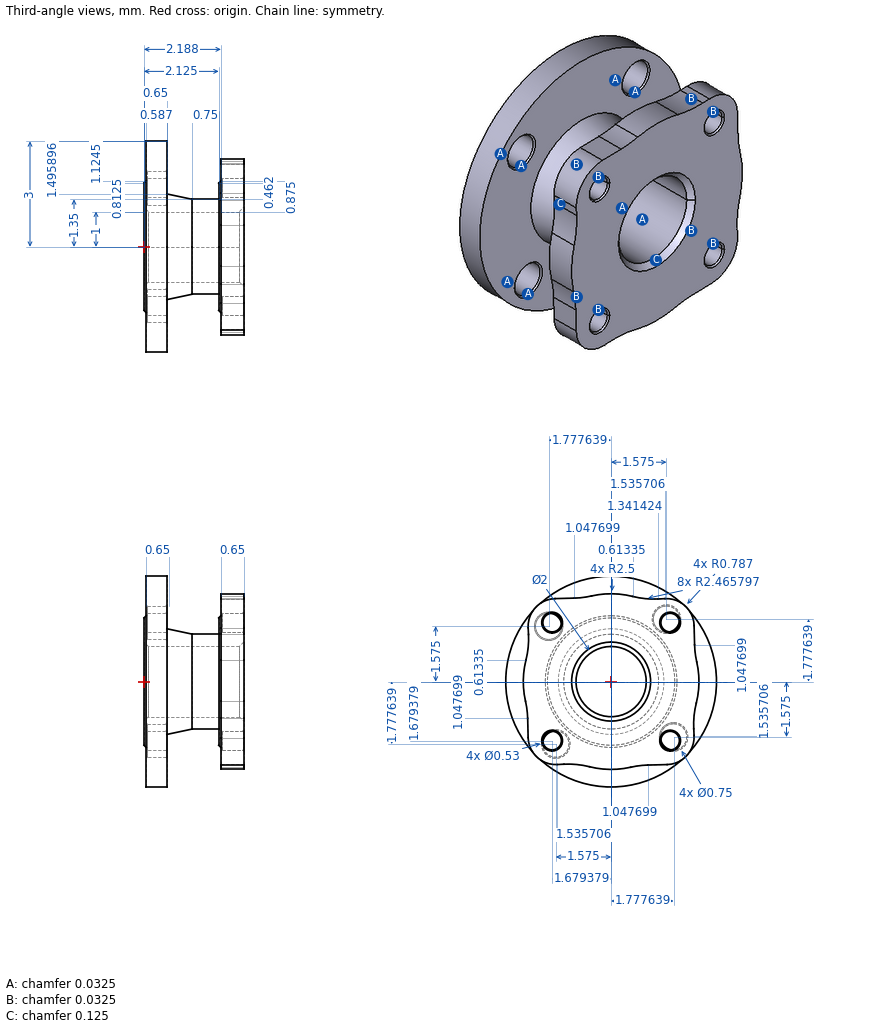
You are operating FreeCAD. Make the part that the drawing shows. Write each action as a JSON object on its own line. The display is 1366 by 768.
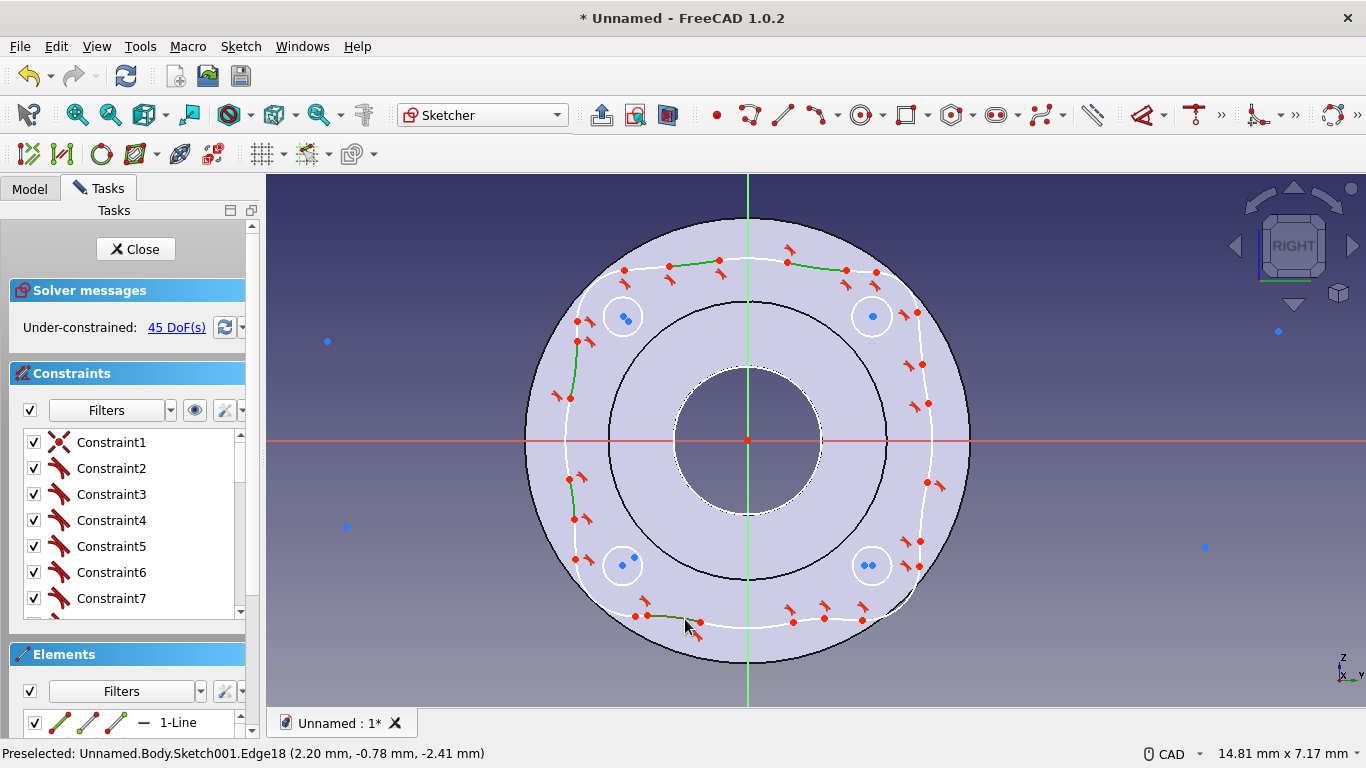
{"action": "scroll", "coordinate": [815, 619], "scroll_direction": "up", "scroll_amount": 2}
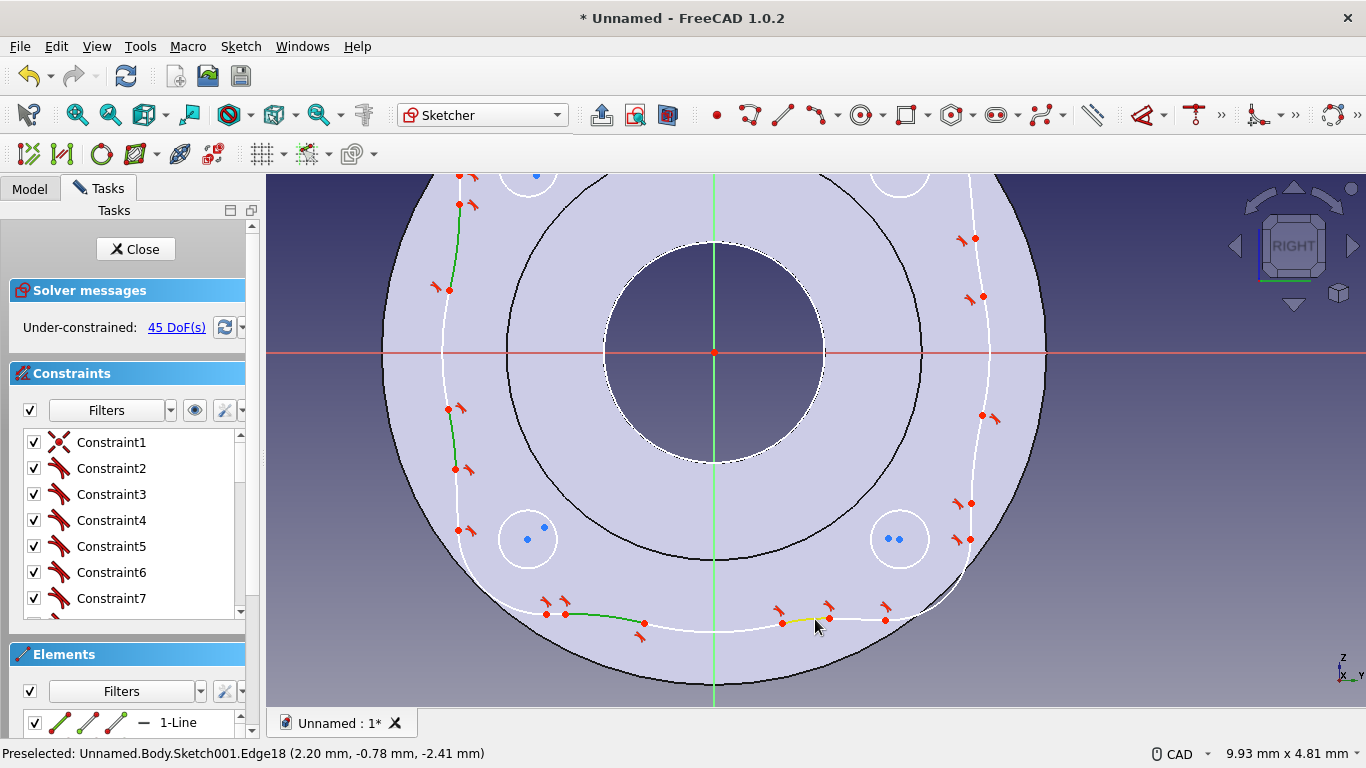
{"action": "left_click", "coordinate": [815, 619]}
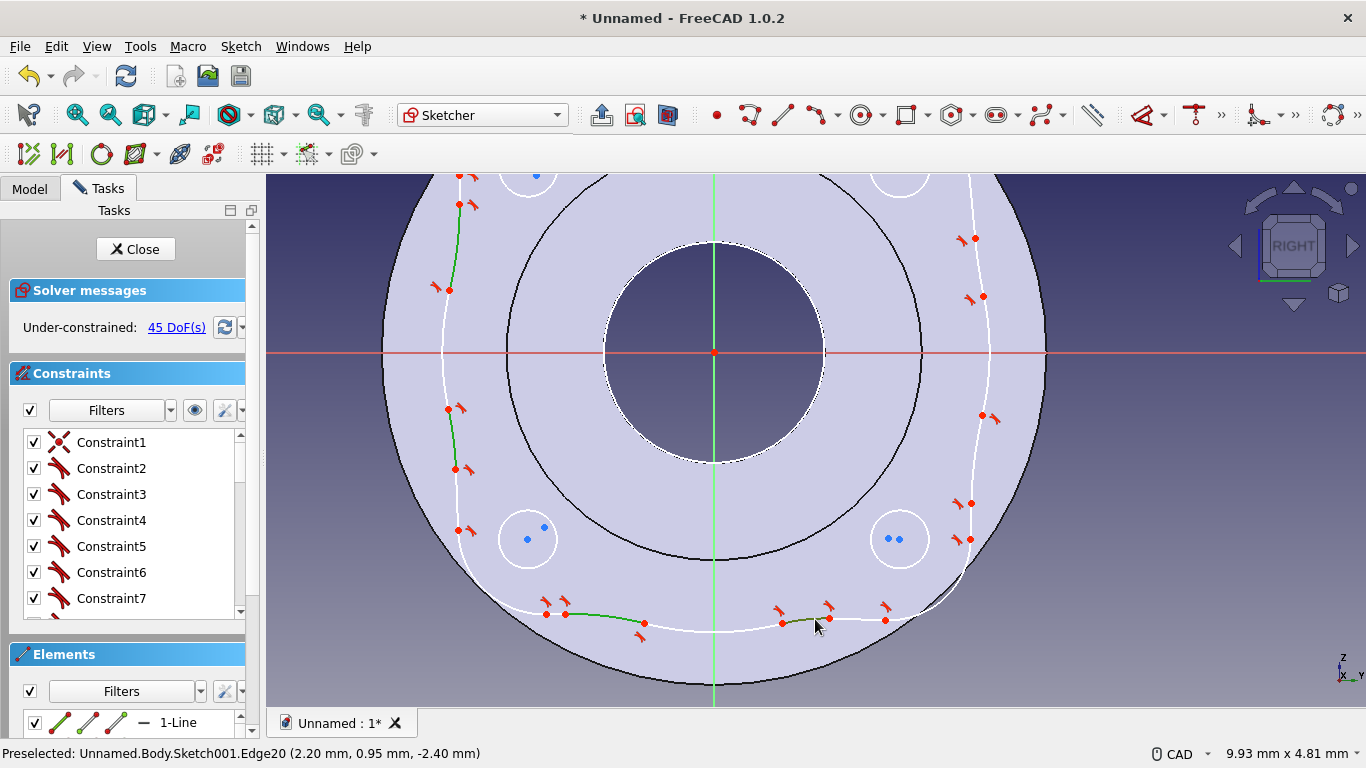
{"action": "left_click", "coordinate": [977, 441]}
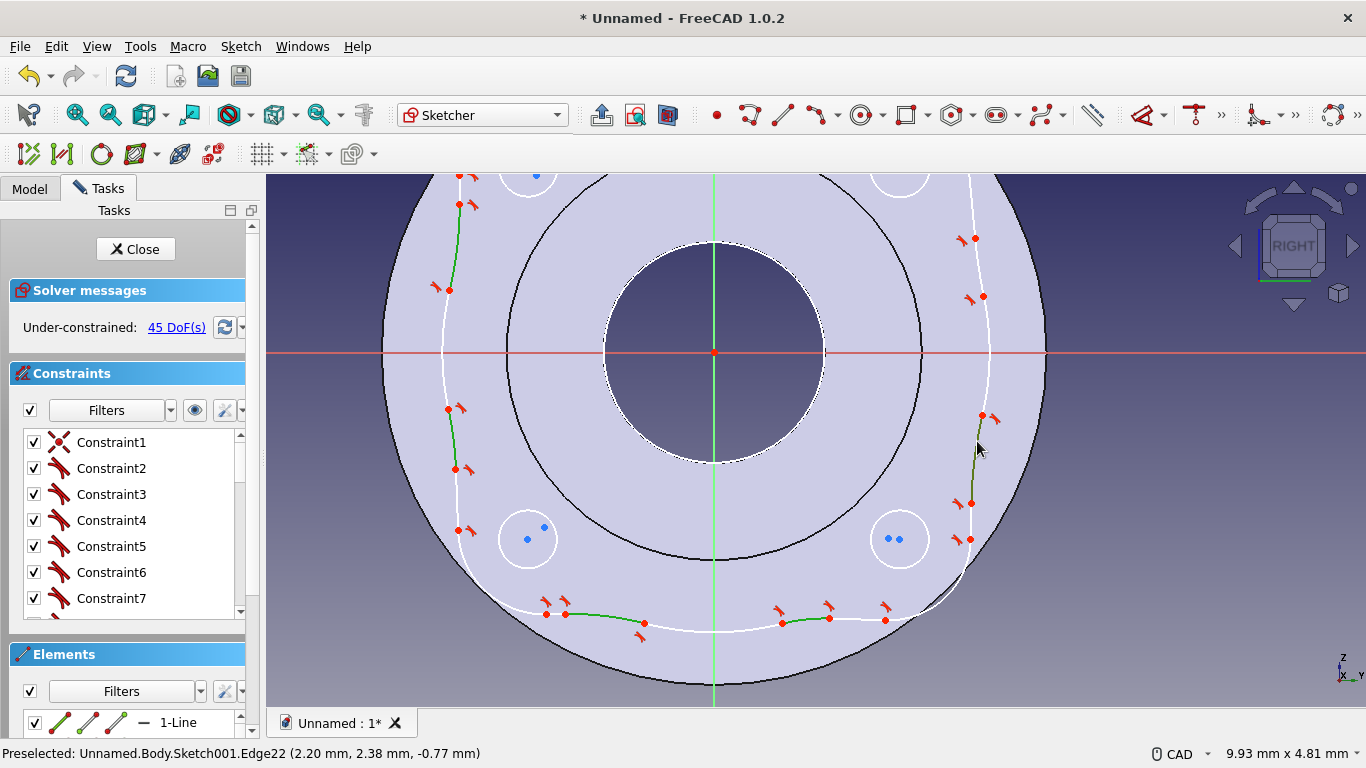
{"action": "left_click", "coordinate": [977, 256]}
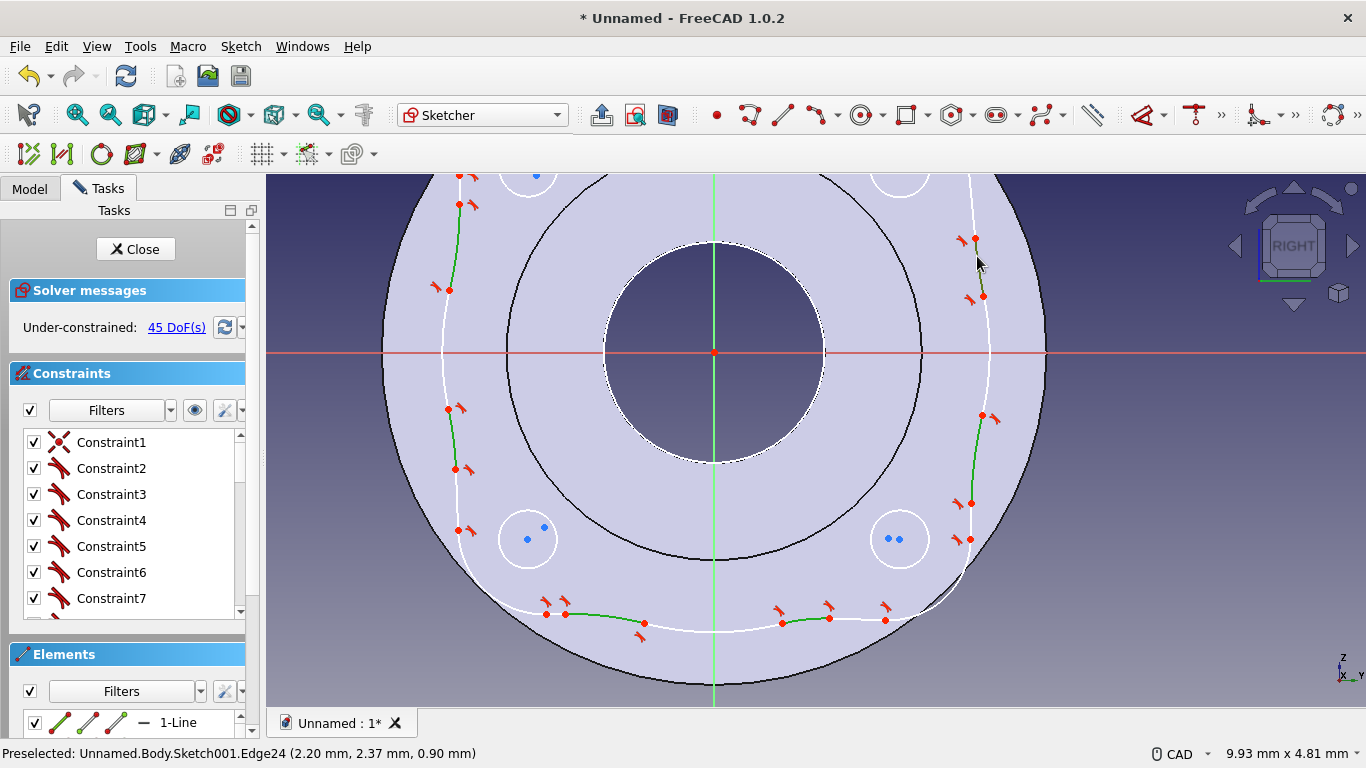
{"action": "key", "text": "e"}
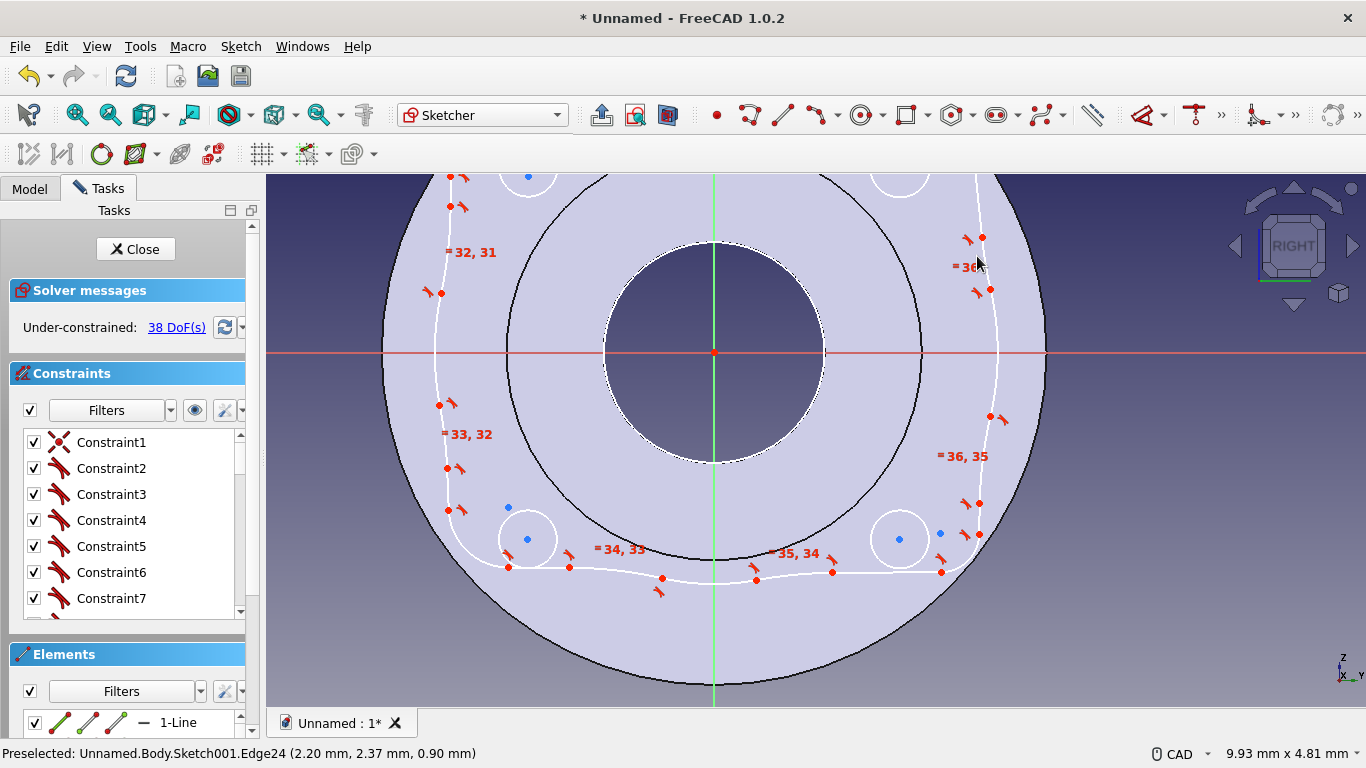
{"action": "scroll", "coordinate": [815, 619], "scroll_direction": "down", "scroll_amount": 2}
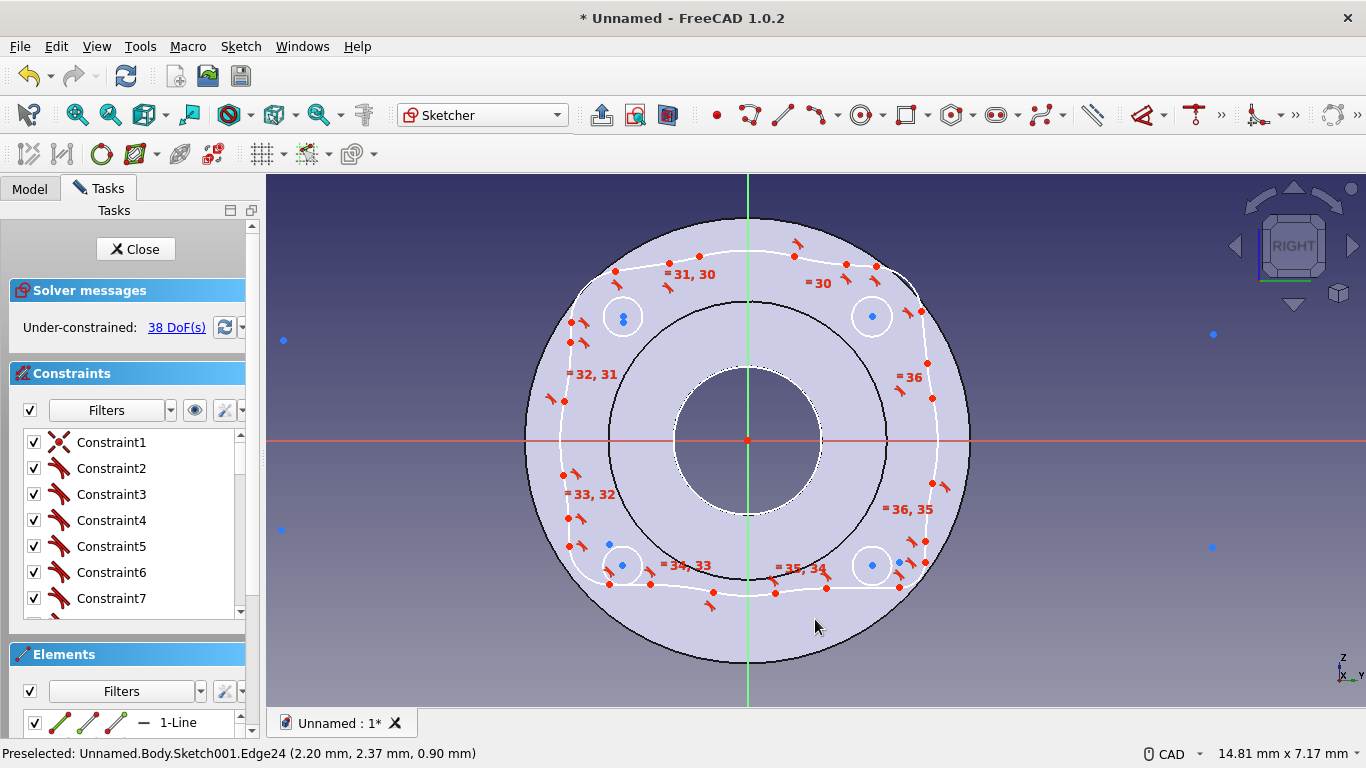
{"action": "left_click", "coordinate": [915, 292]}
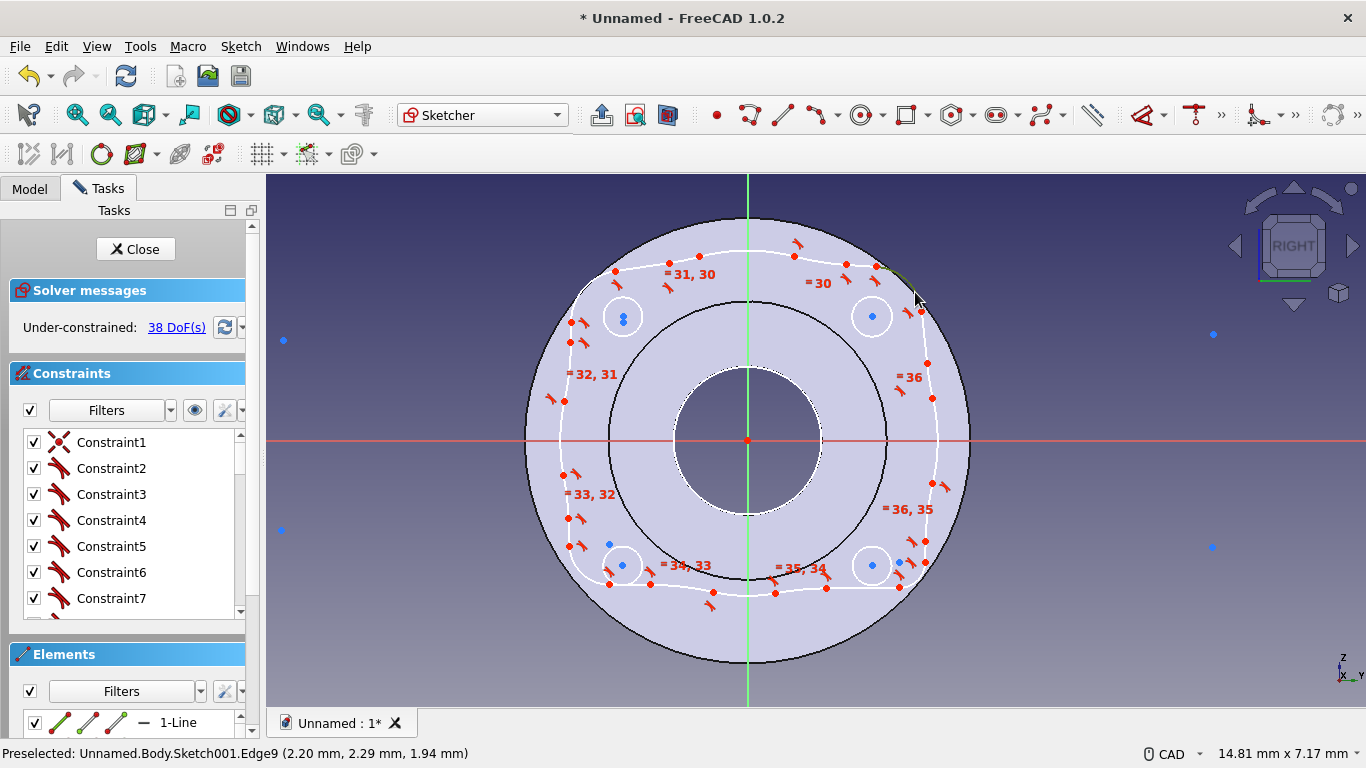
{"action": "left_click", "coordinate": [595, 279]}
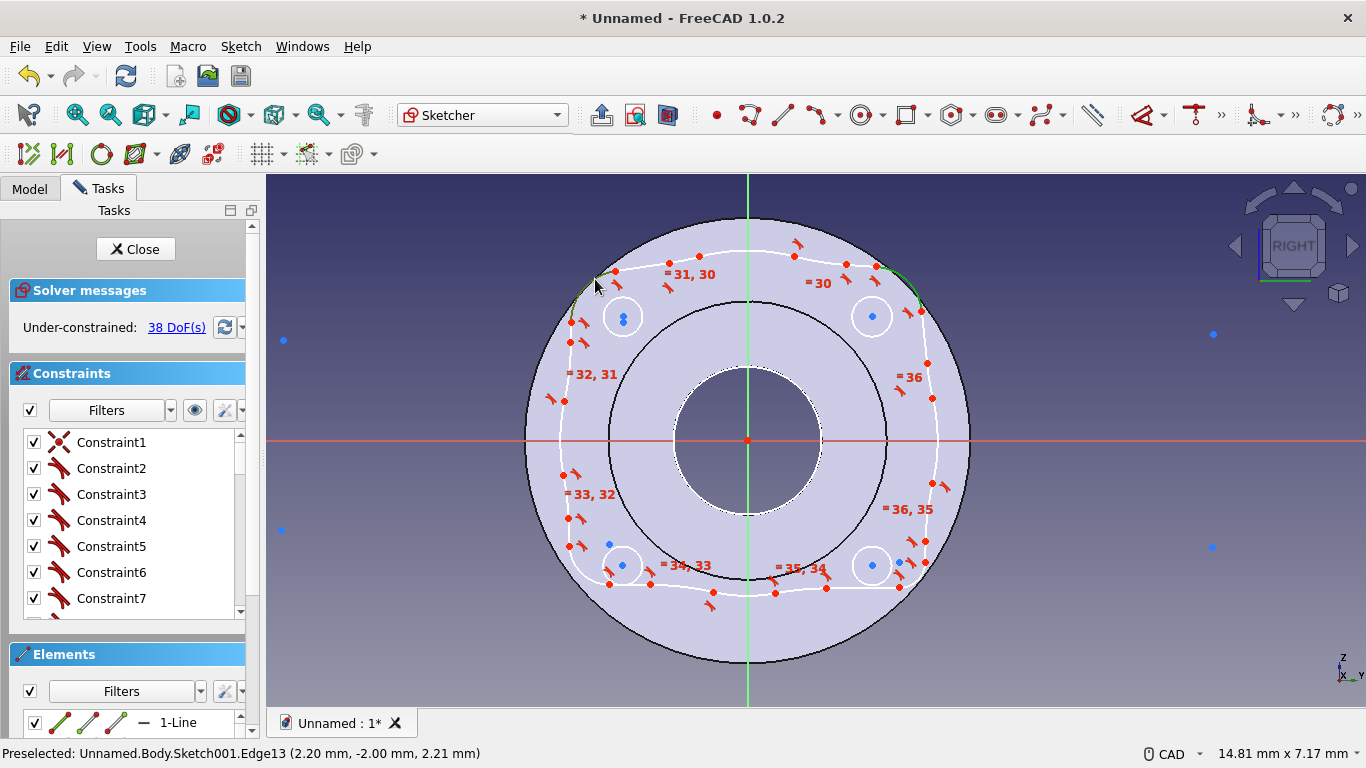
{"action": "left_click", "coordinate": [575, 564]}